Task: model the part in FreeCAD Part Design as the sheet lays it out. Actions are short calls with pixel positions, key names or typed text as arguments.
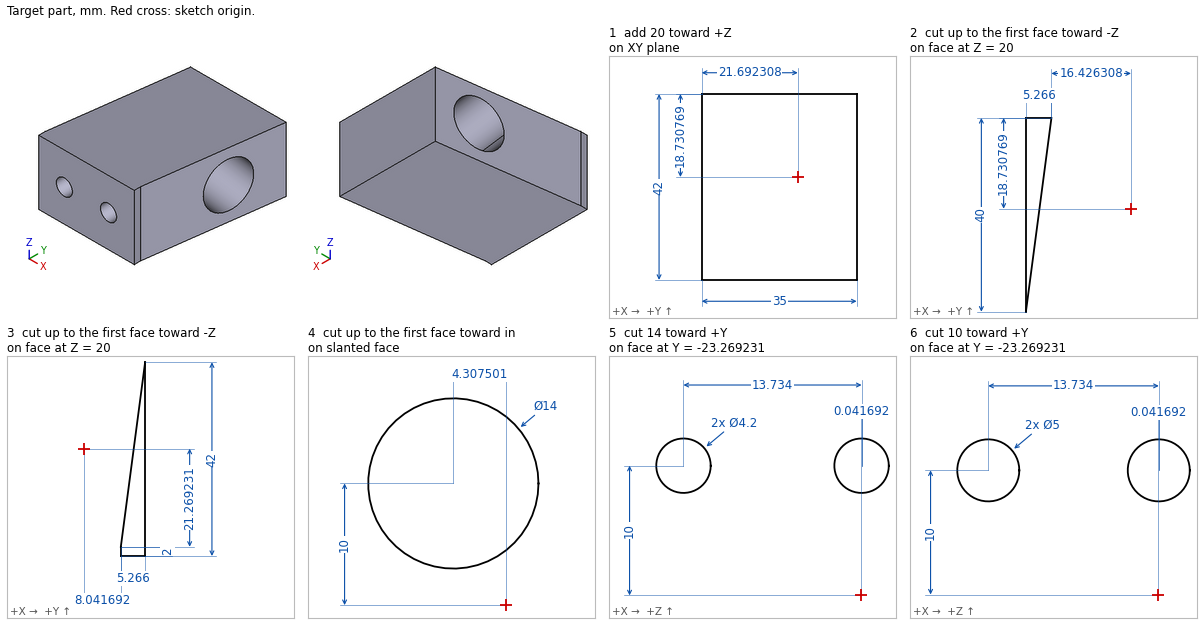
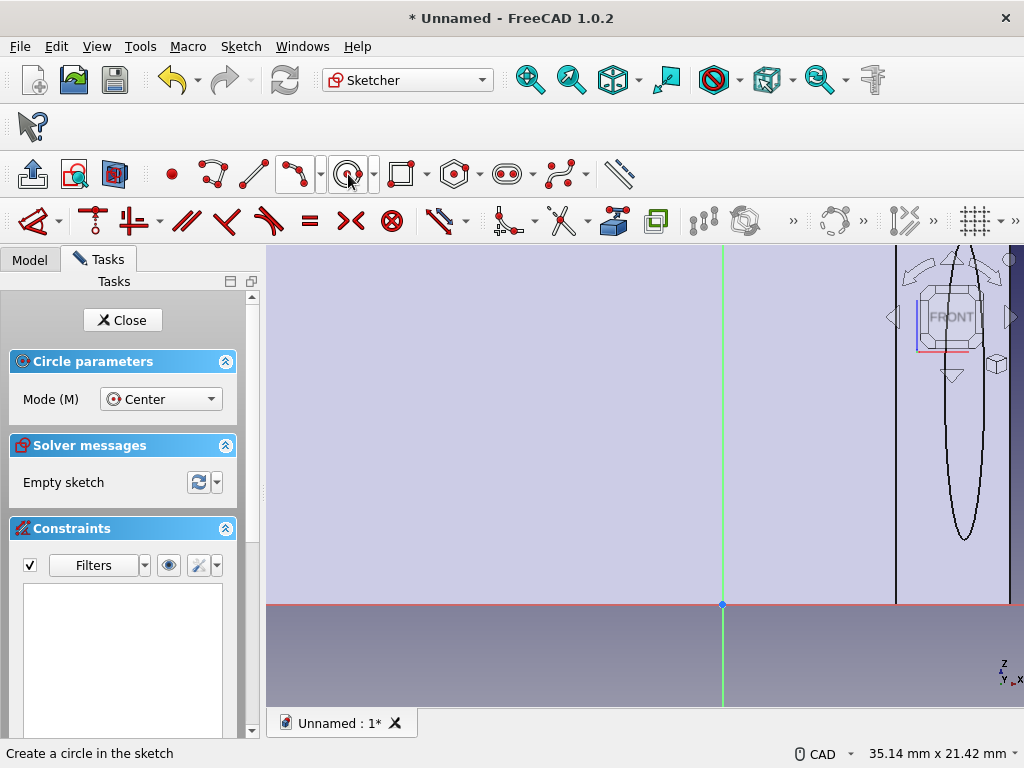
click(427, 389)
click(459, 357)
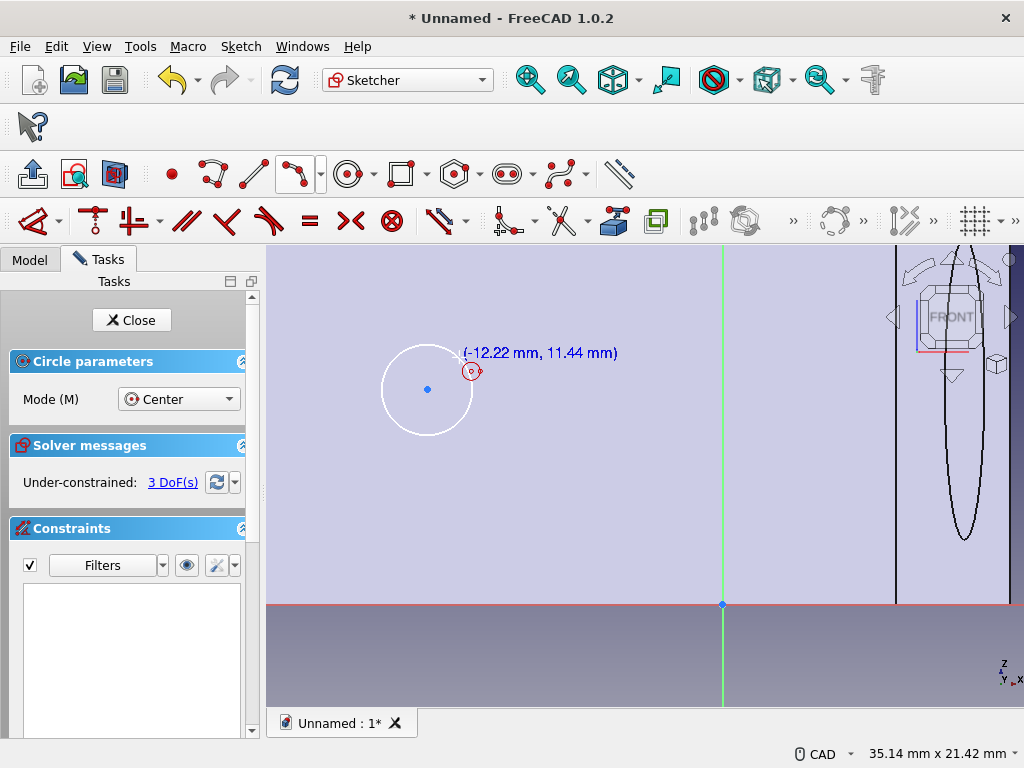
scroll(723, 389, up, 15)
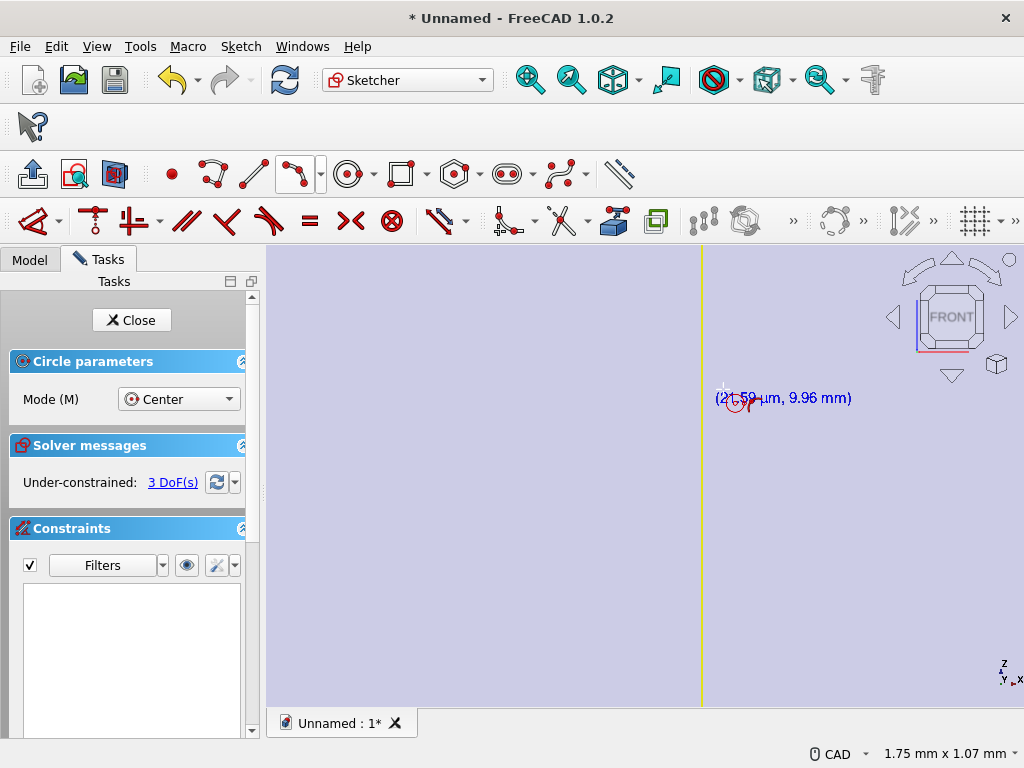
click(720, 384)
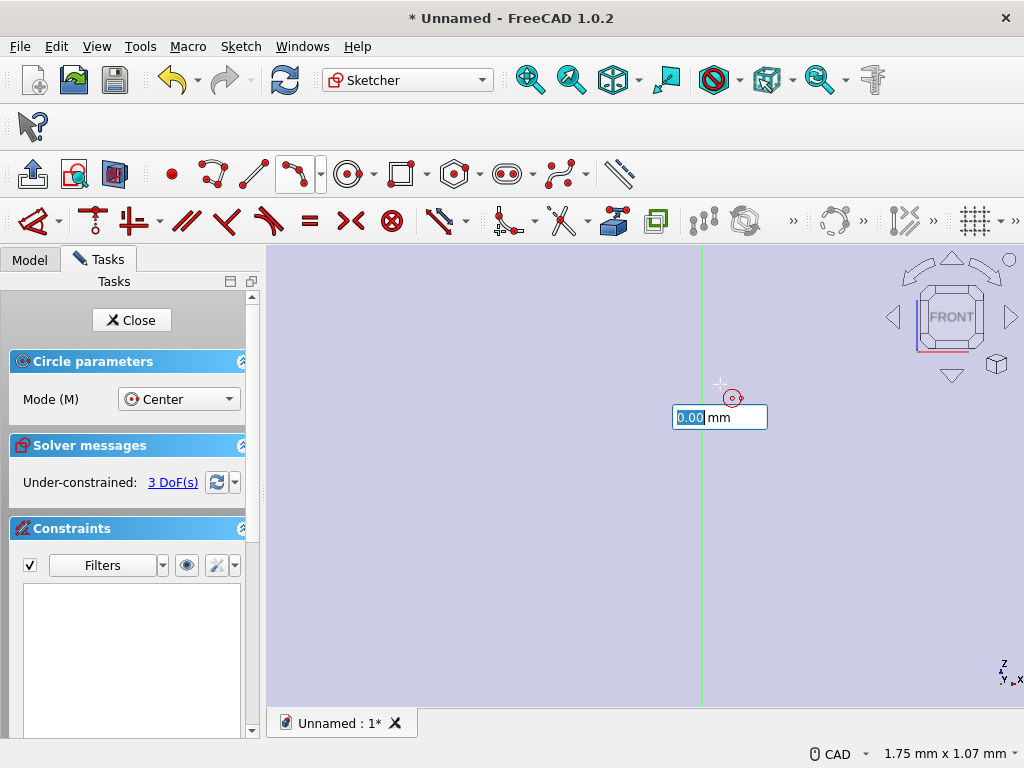
scroll(725, 391, down, 15)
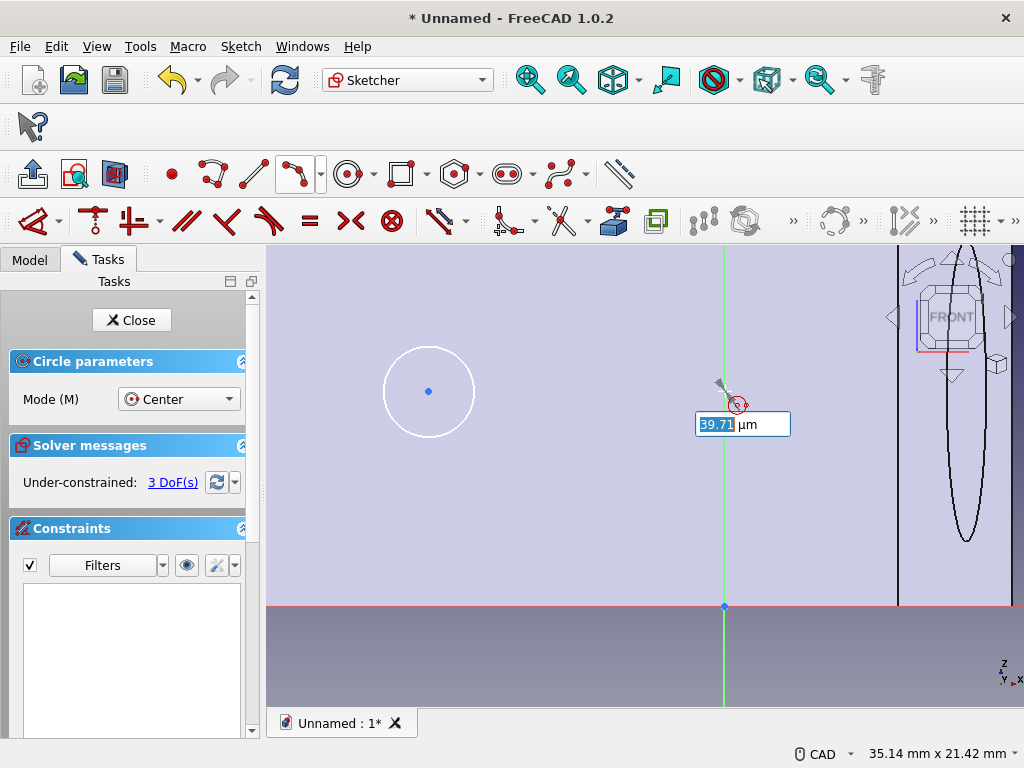
click(757, 359)
key(Escape)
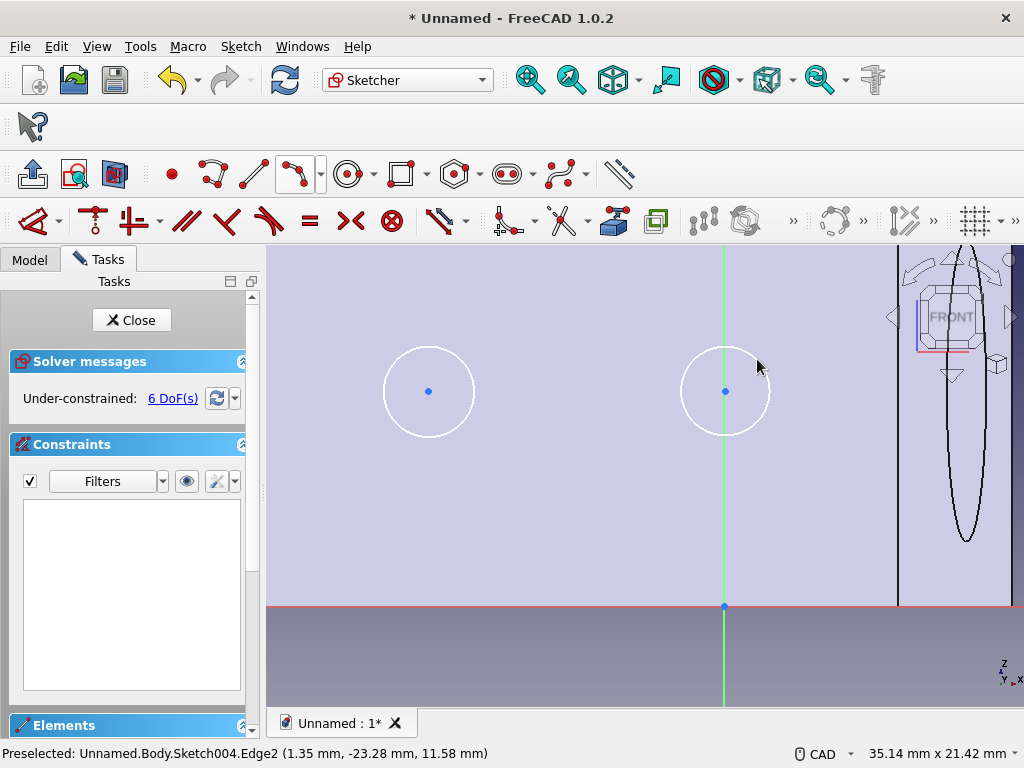
click(461, 360)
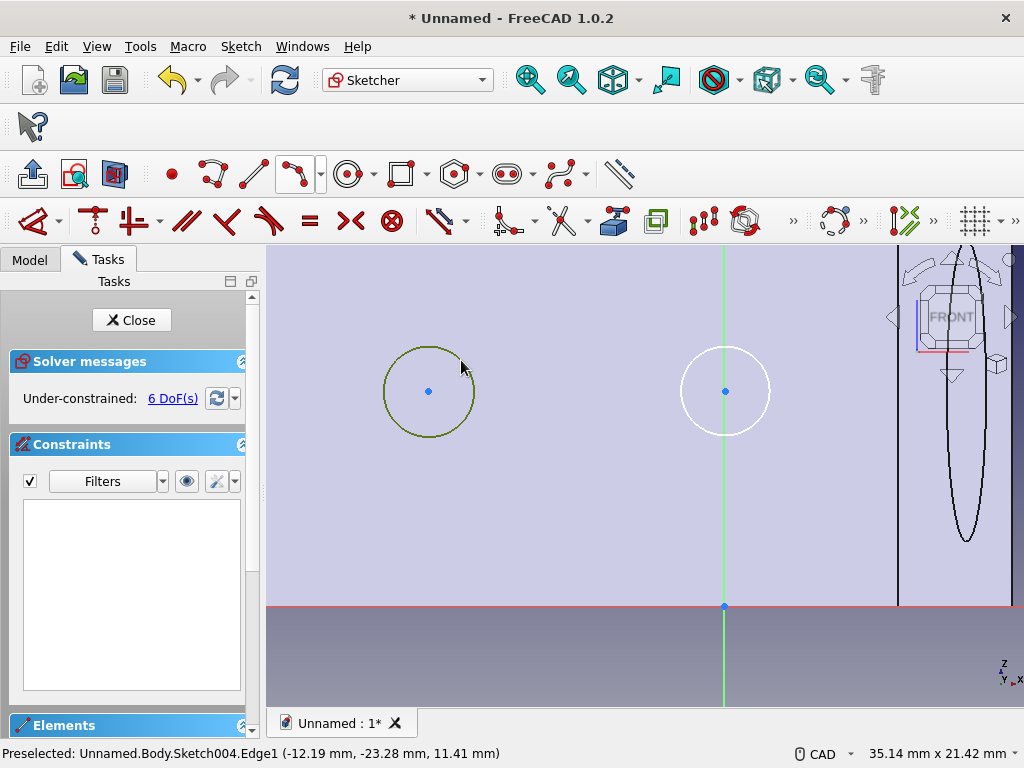
click(757, 360)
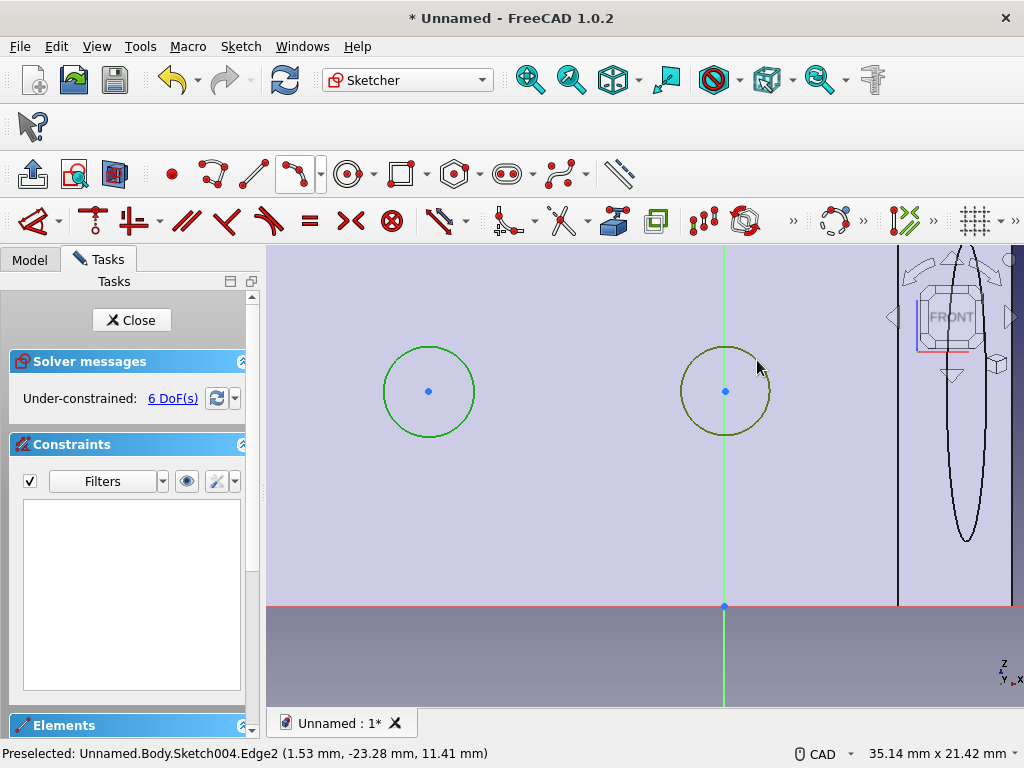
click(310, 222)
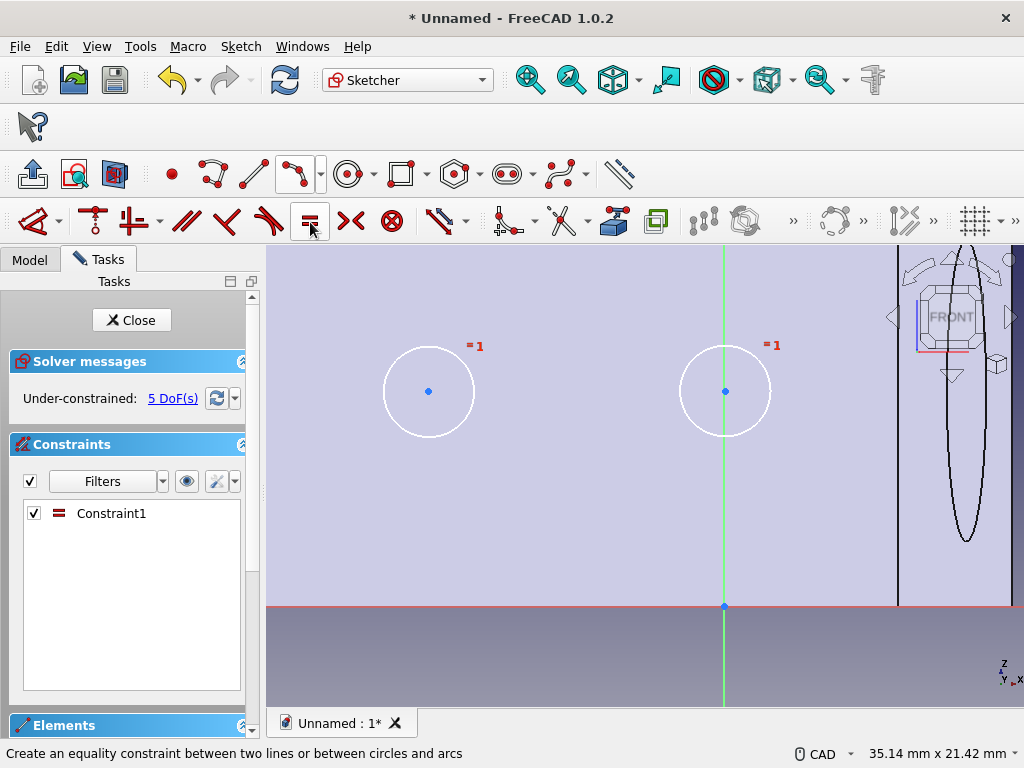
click(429, 392)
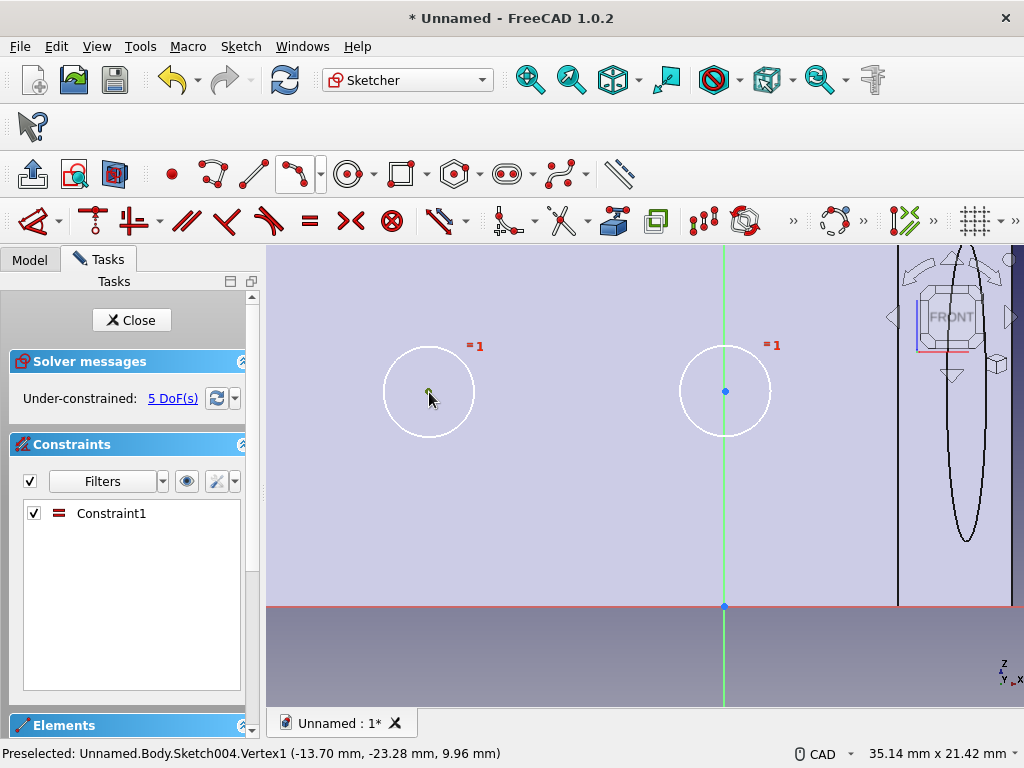
click(725, 391)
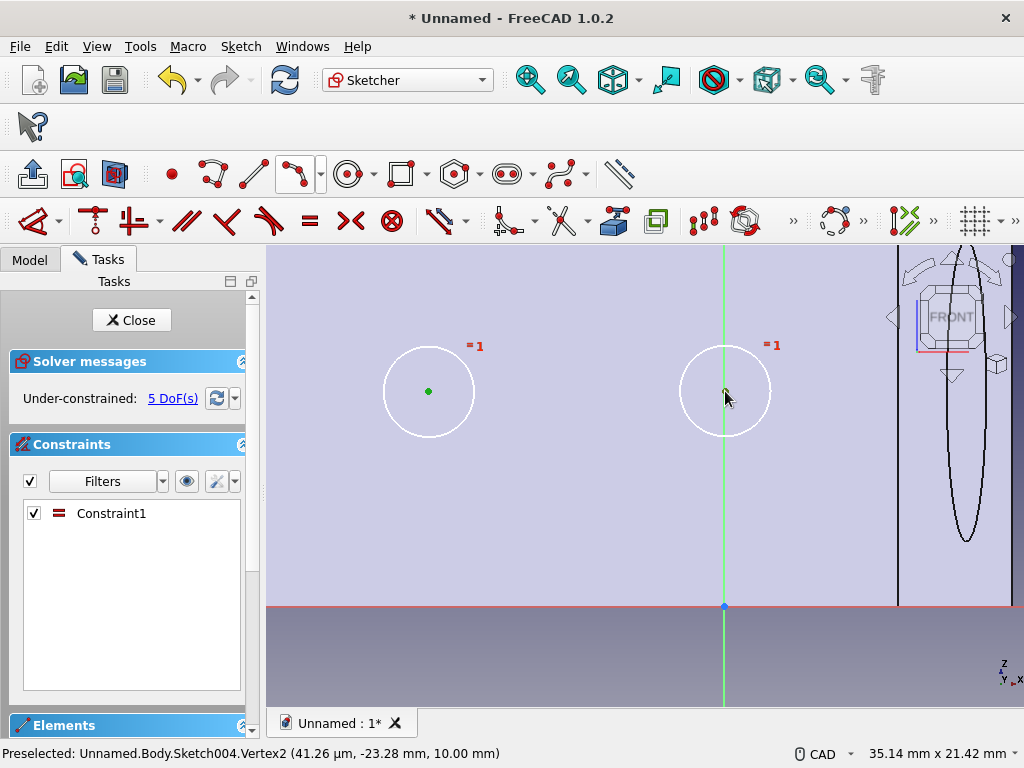
click(160, 222)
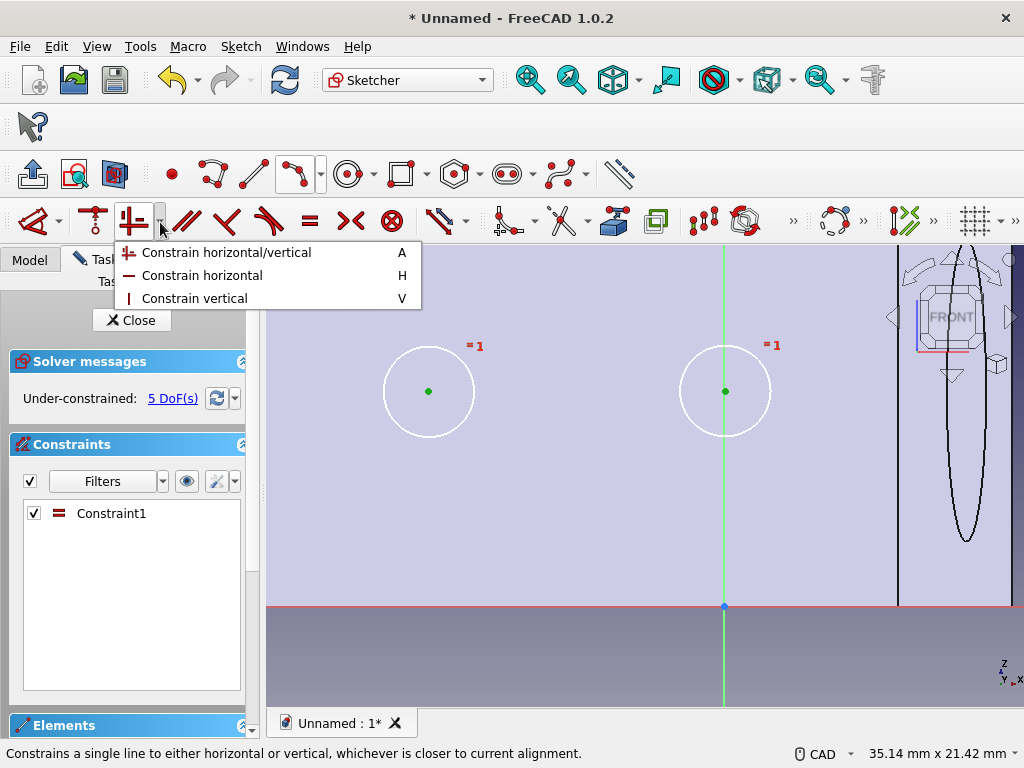
click(268, 276)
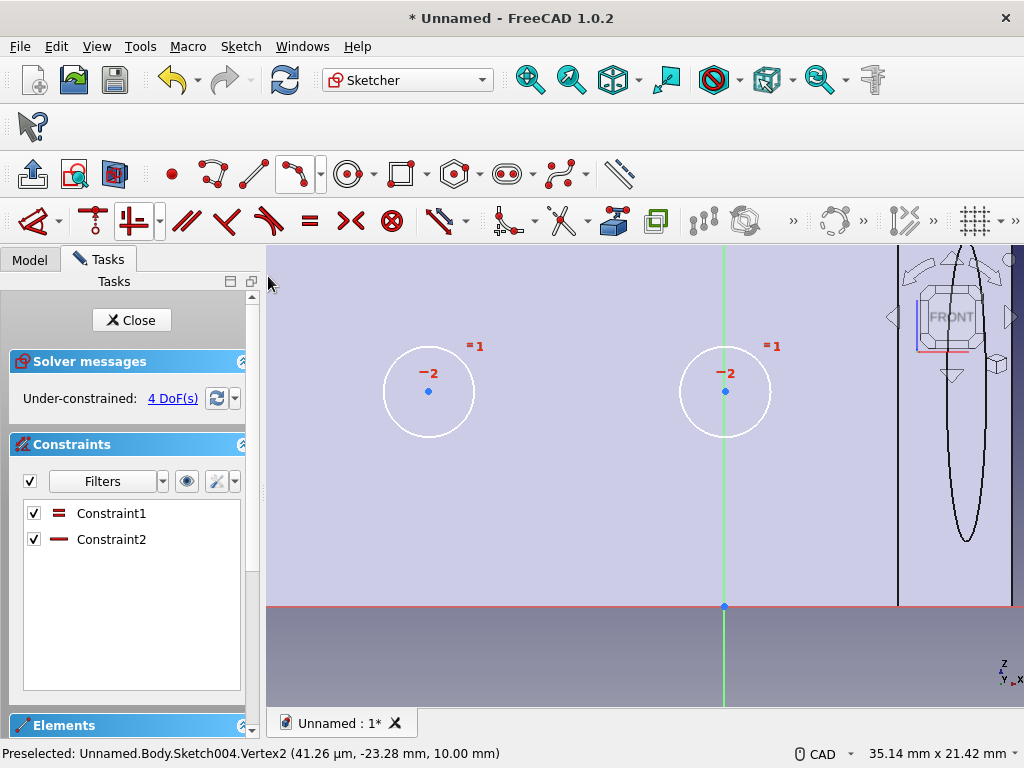
click(32, 222)